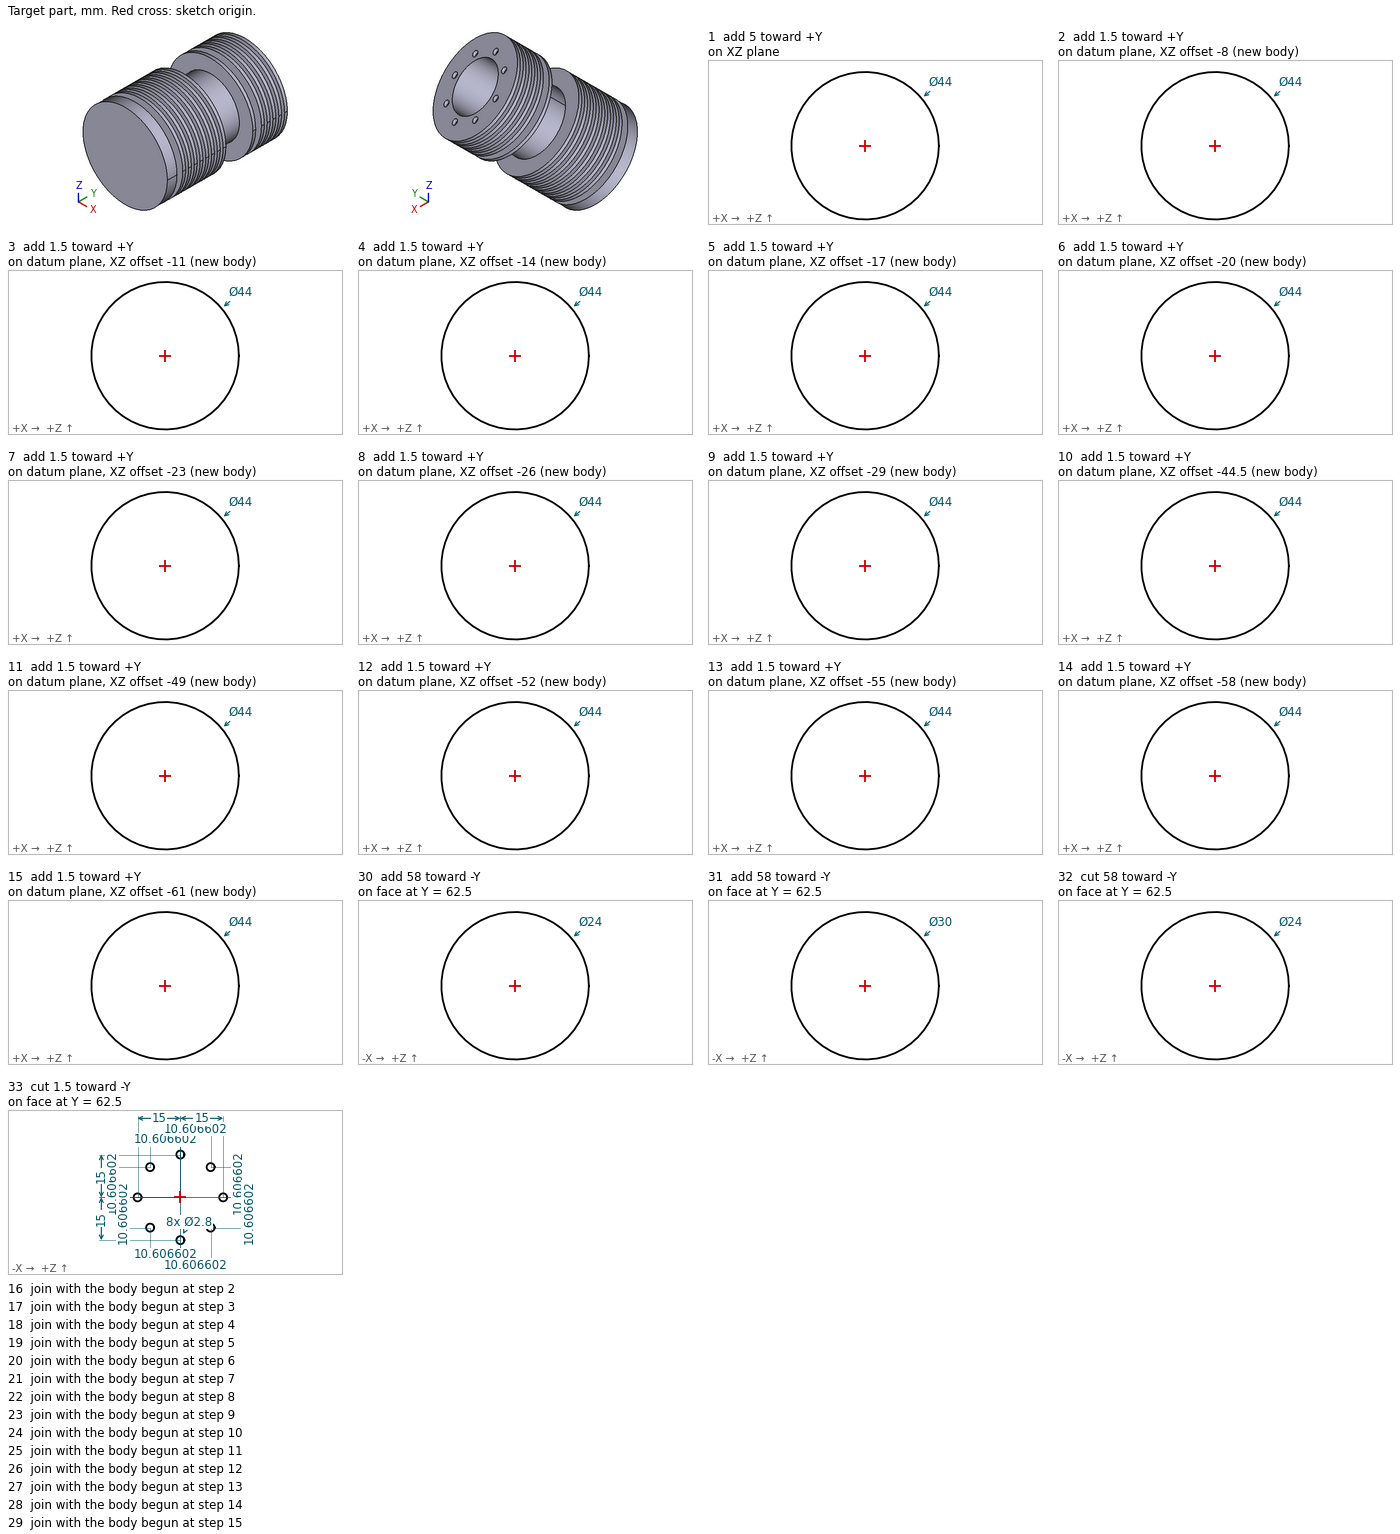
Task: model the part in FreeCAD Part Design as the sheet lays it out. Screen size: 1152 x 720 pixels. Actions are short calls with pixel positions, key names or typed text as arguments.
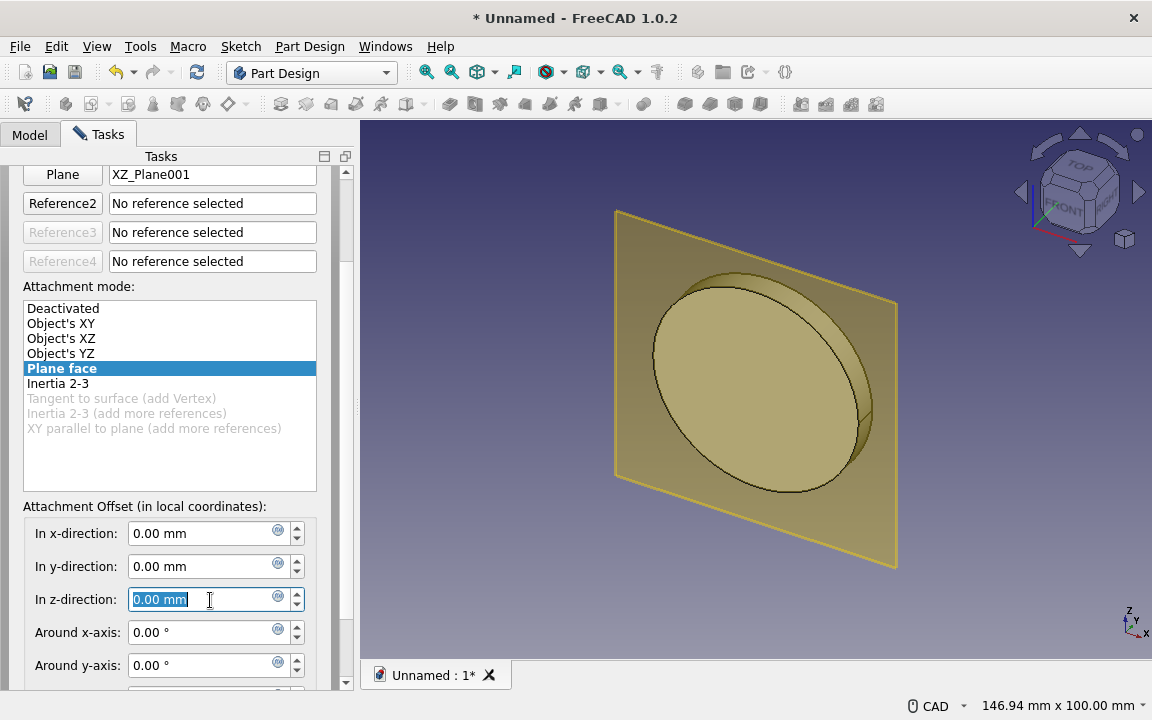
text(-8)
key(Tab)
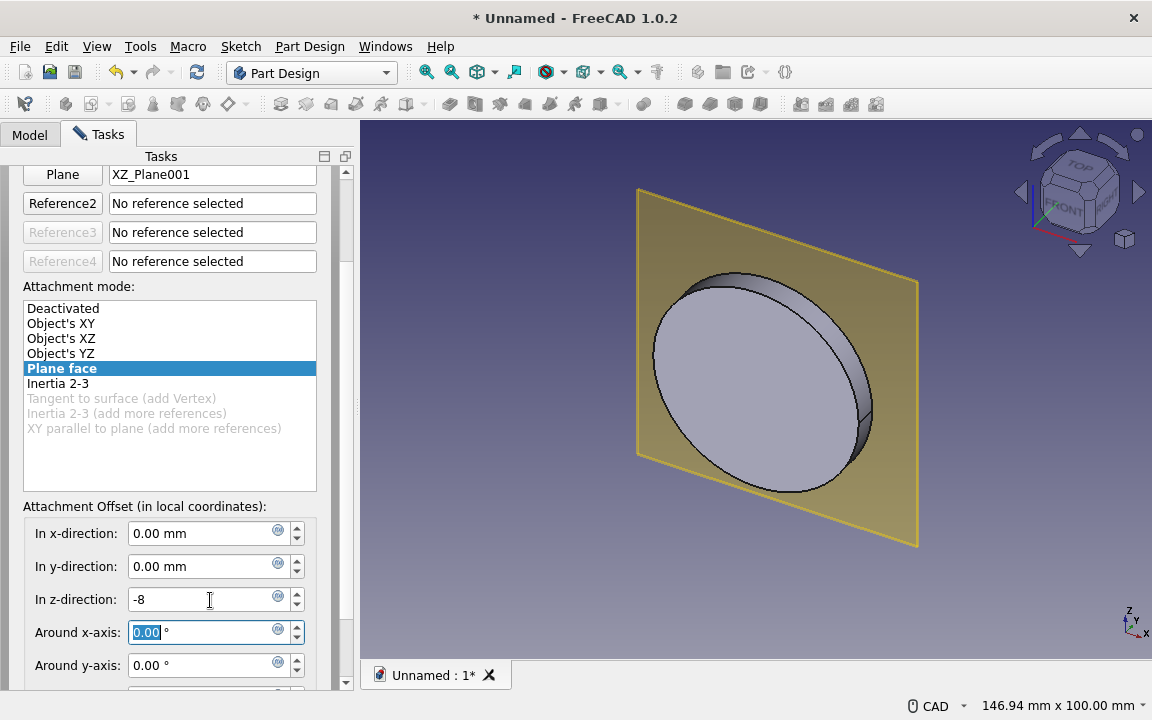
scroll(346, 428, up, 3)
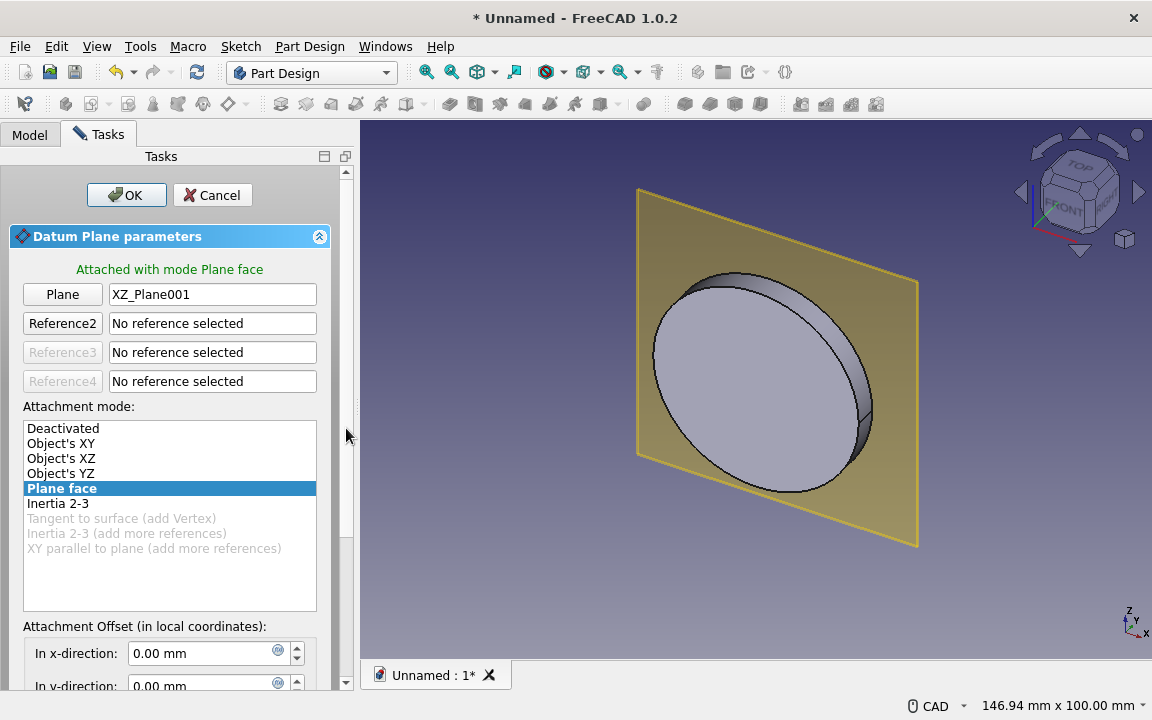
click(127, 195)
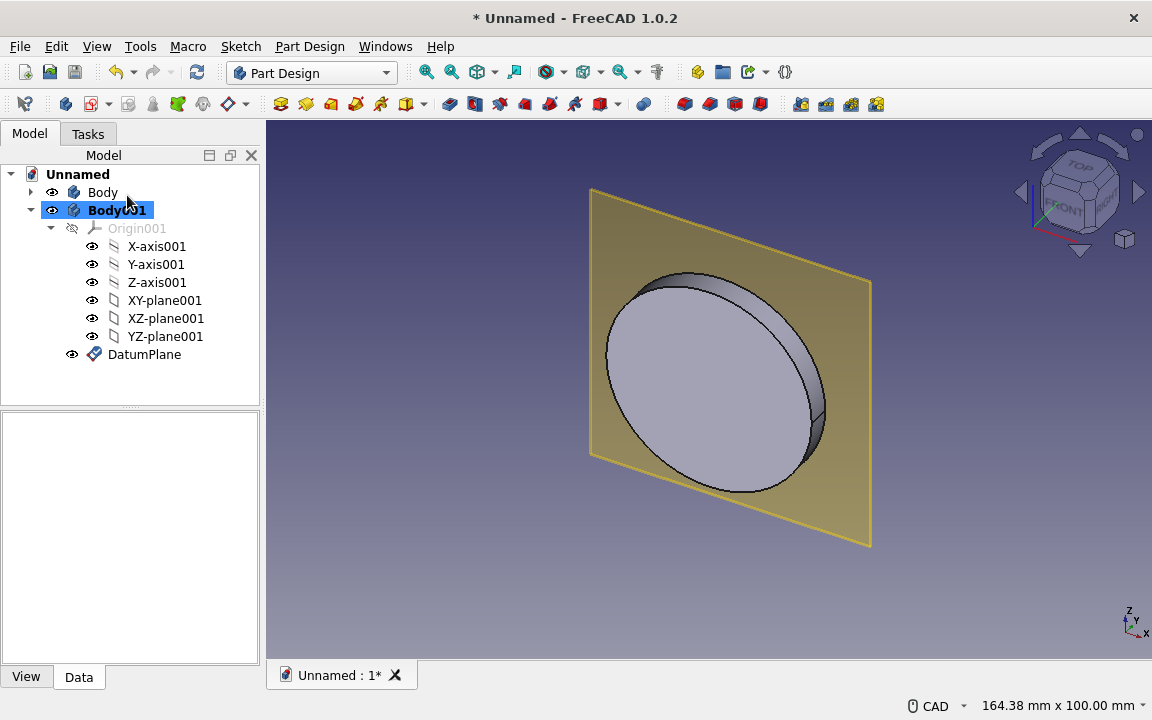
click(117, 354)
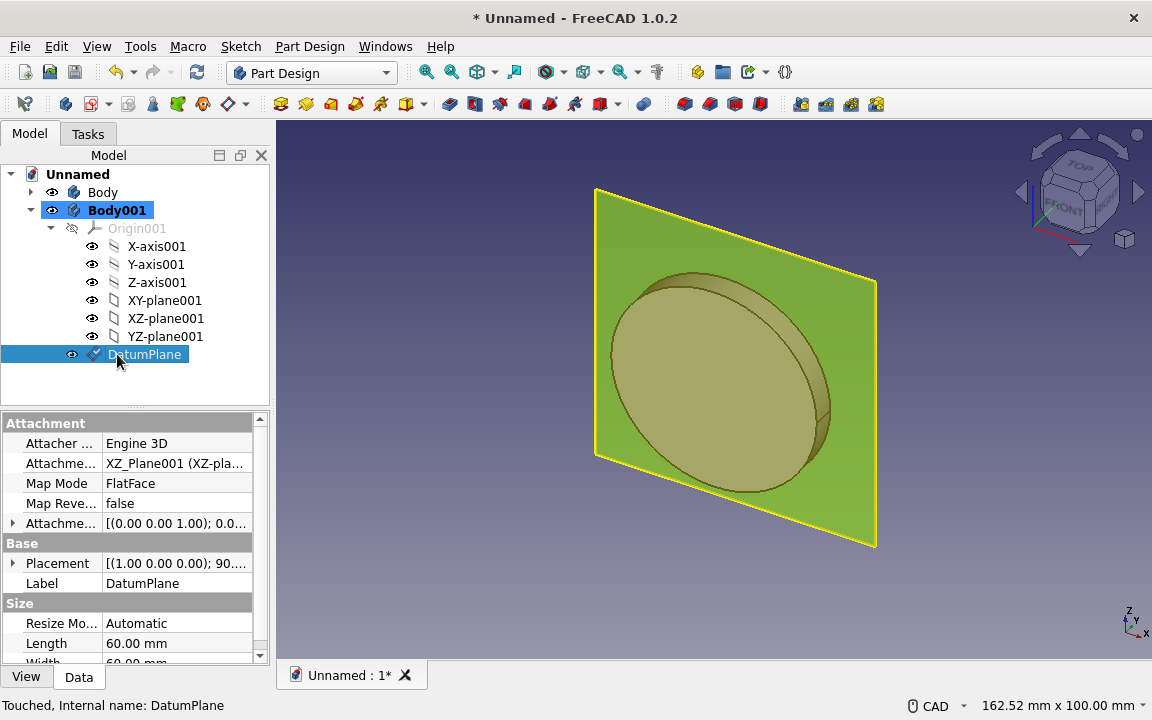
click(90, 104)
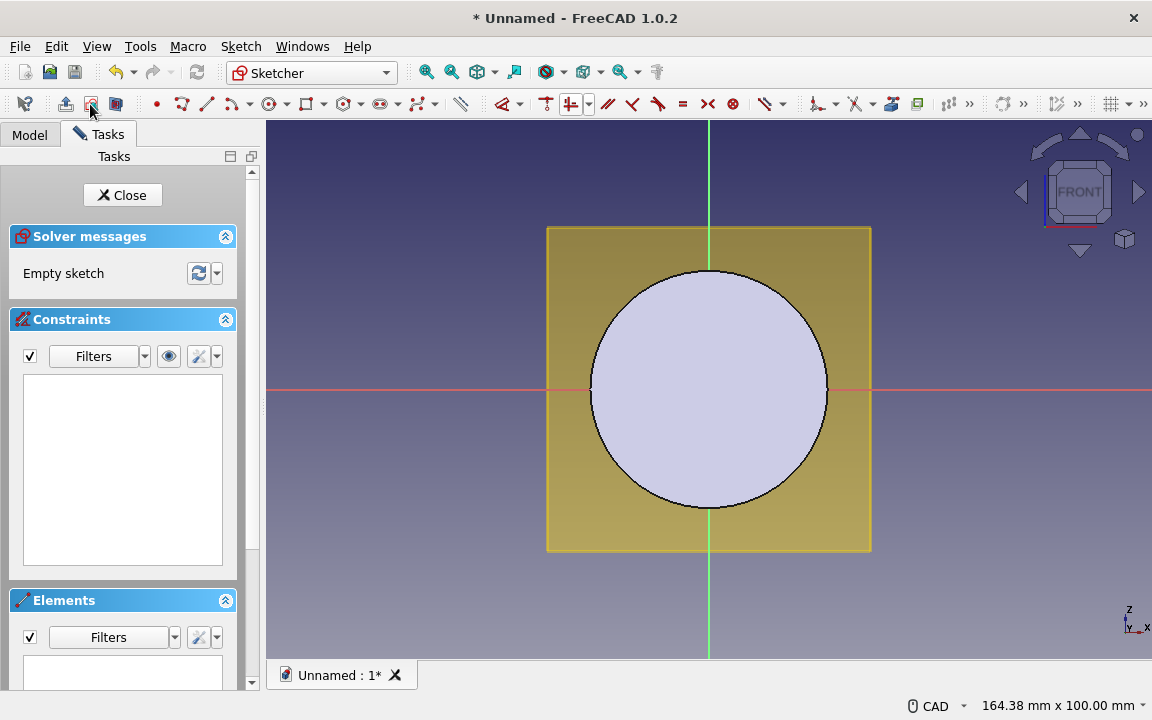
scroll(848, 390, up, 2)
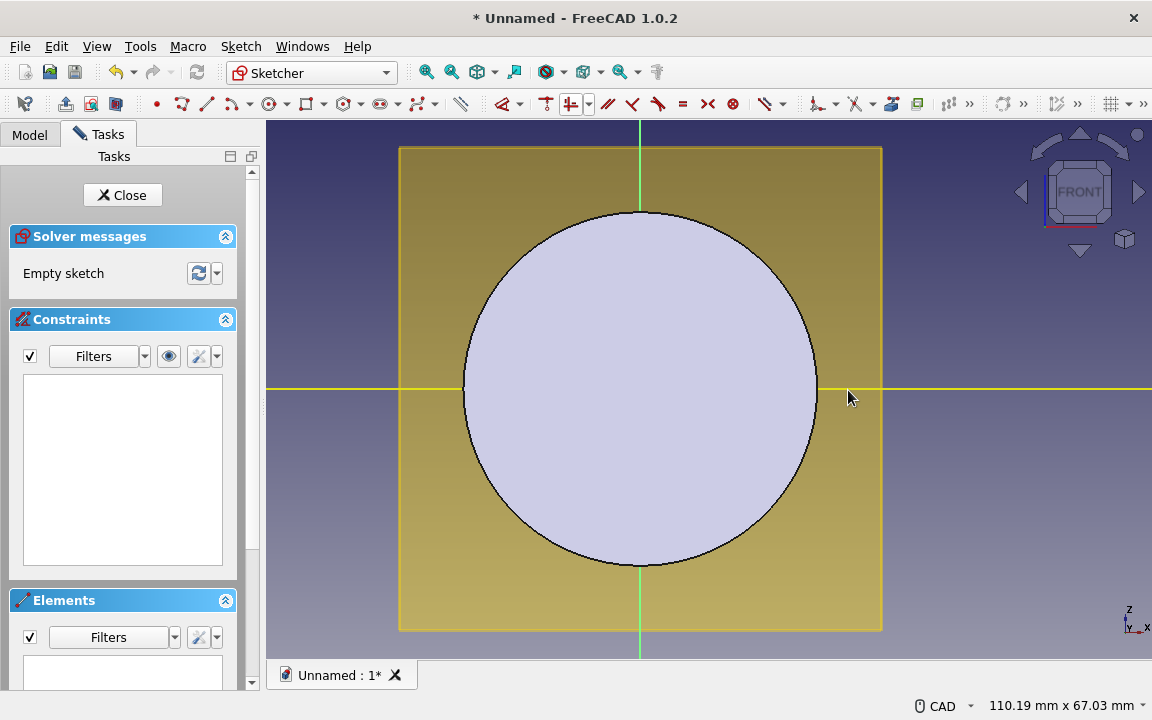
key(g)
key(c)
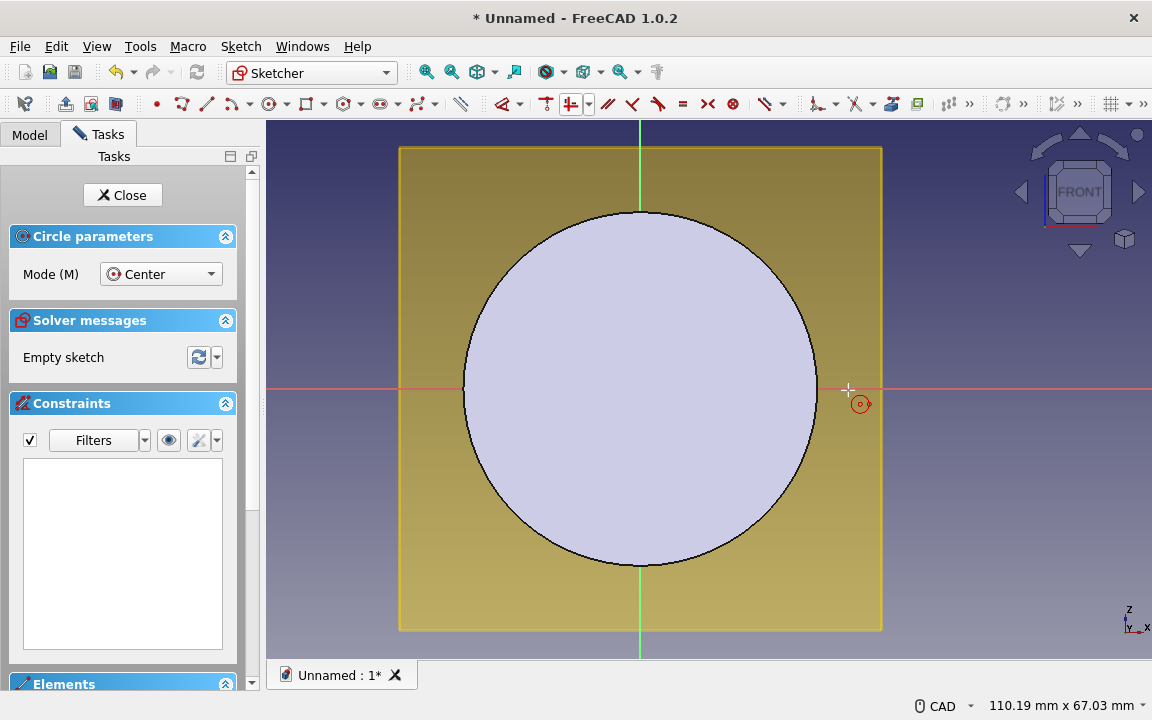
click(640, 389)
click(765, 264)
key(Escape)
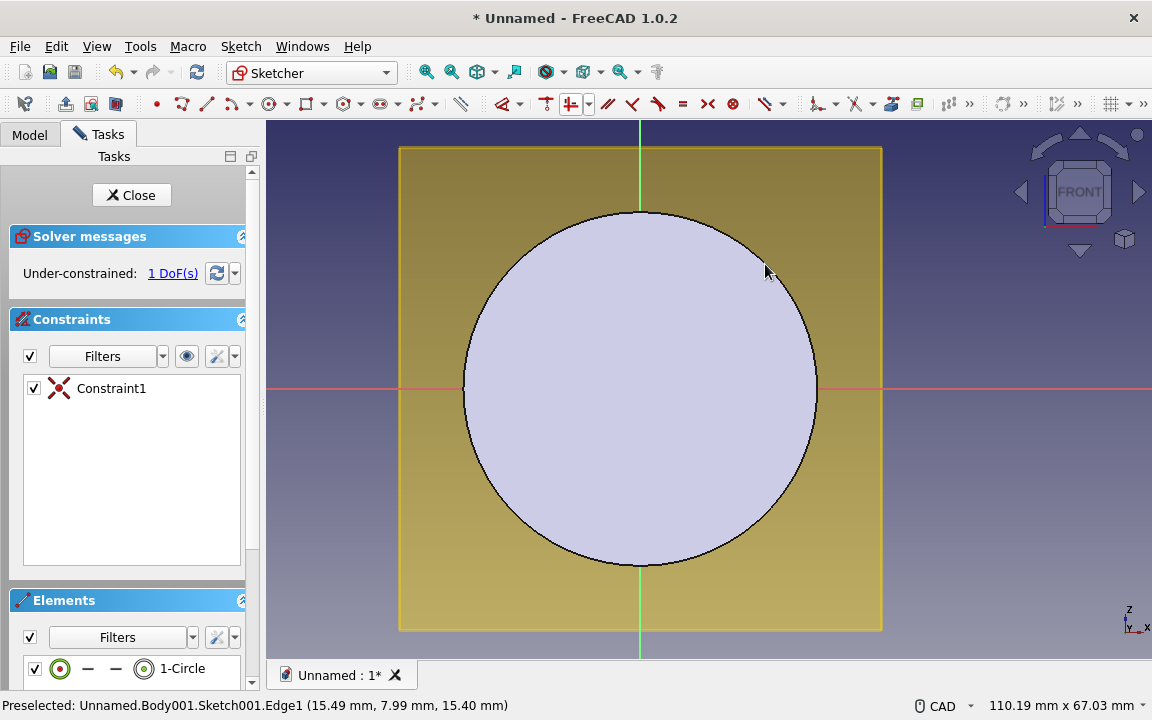
click(764, 264)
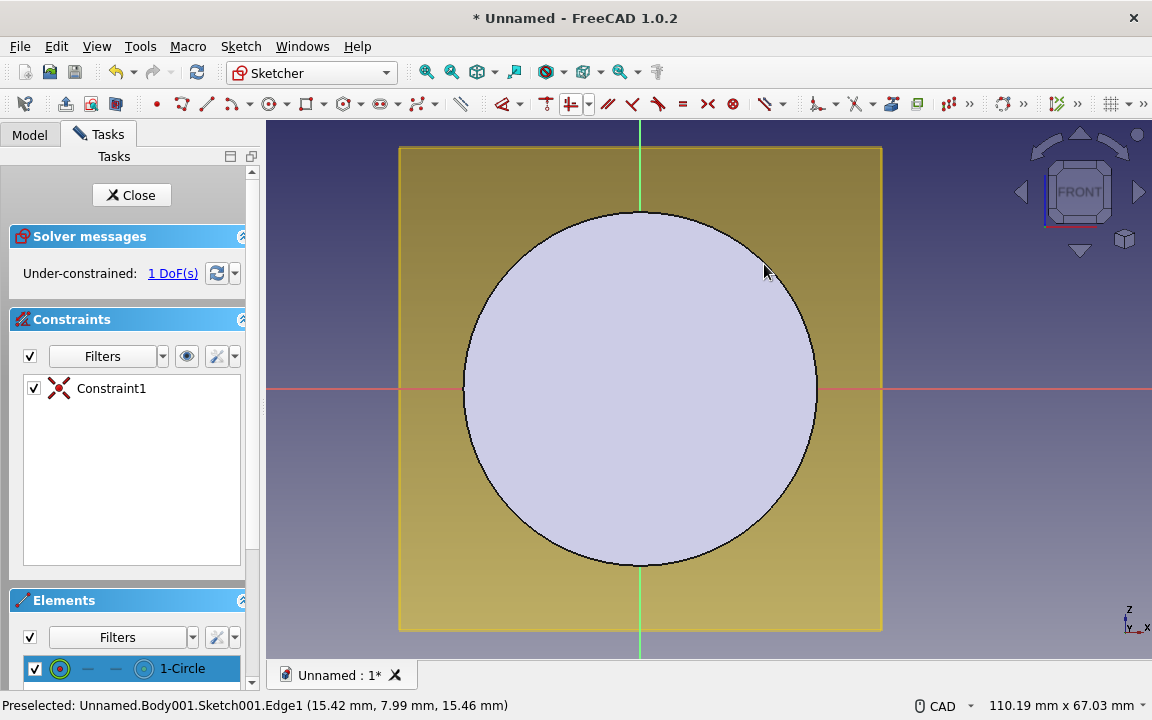
key(k)
key(o)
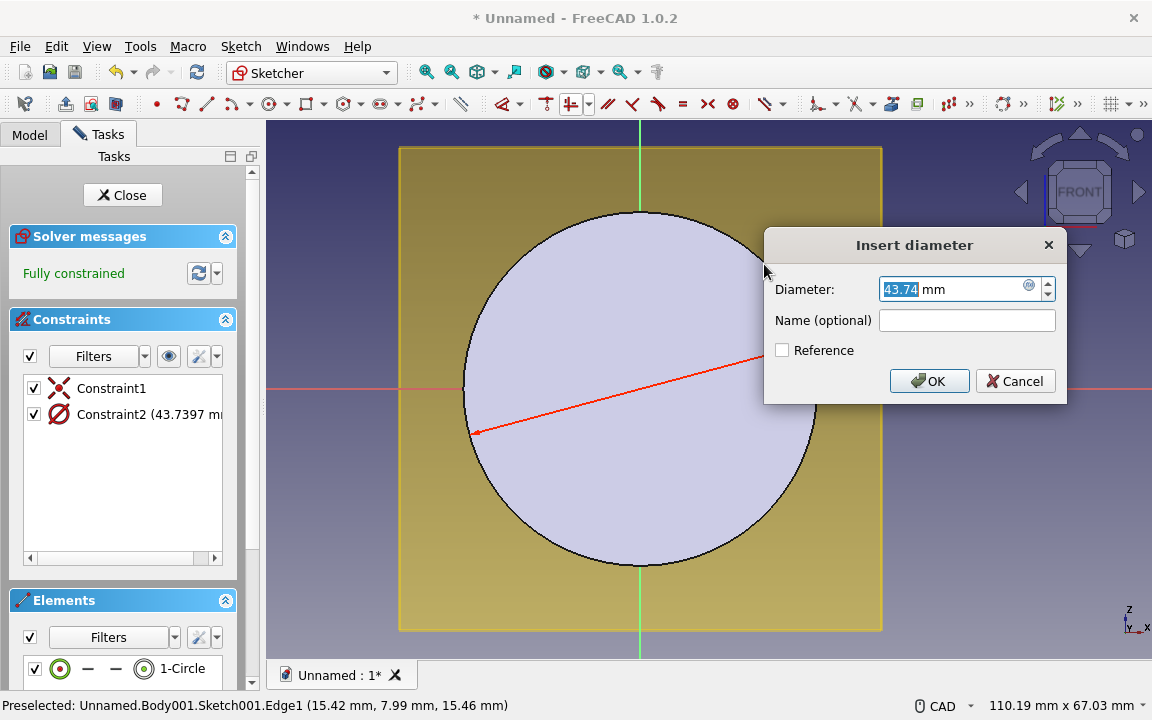
text(44)
key(Return)